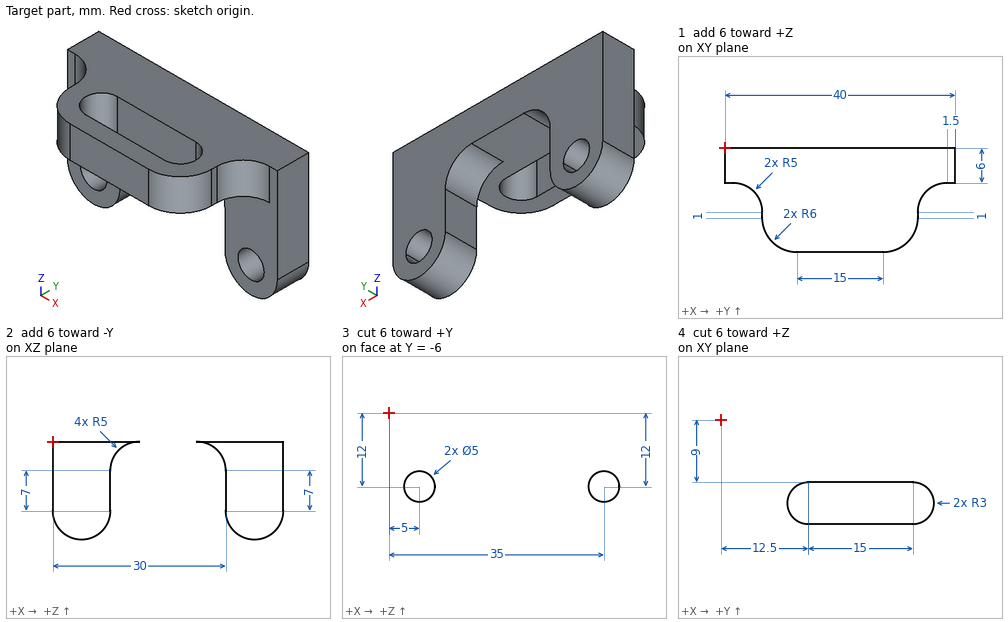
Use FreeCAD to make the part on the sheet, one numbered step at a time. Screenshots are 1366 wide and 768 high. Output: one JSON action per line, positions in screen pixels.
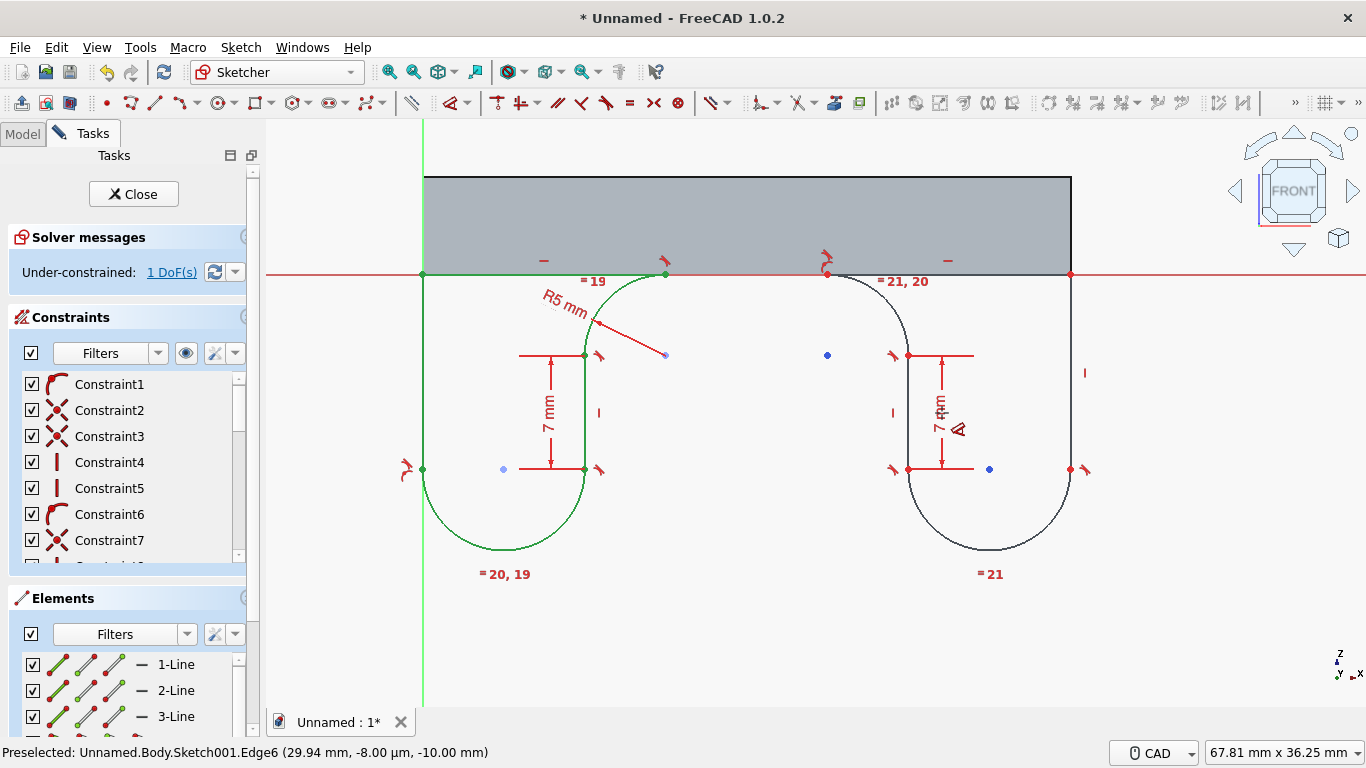
{"action": "left_click", "coordinate": [908, 469]}
{"action": "left_click", "coordinate": [665, 241]}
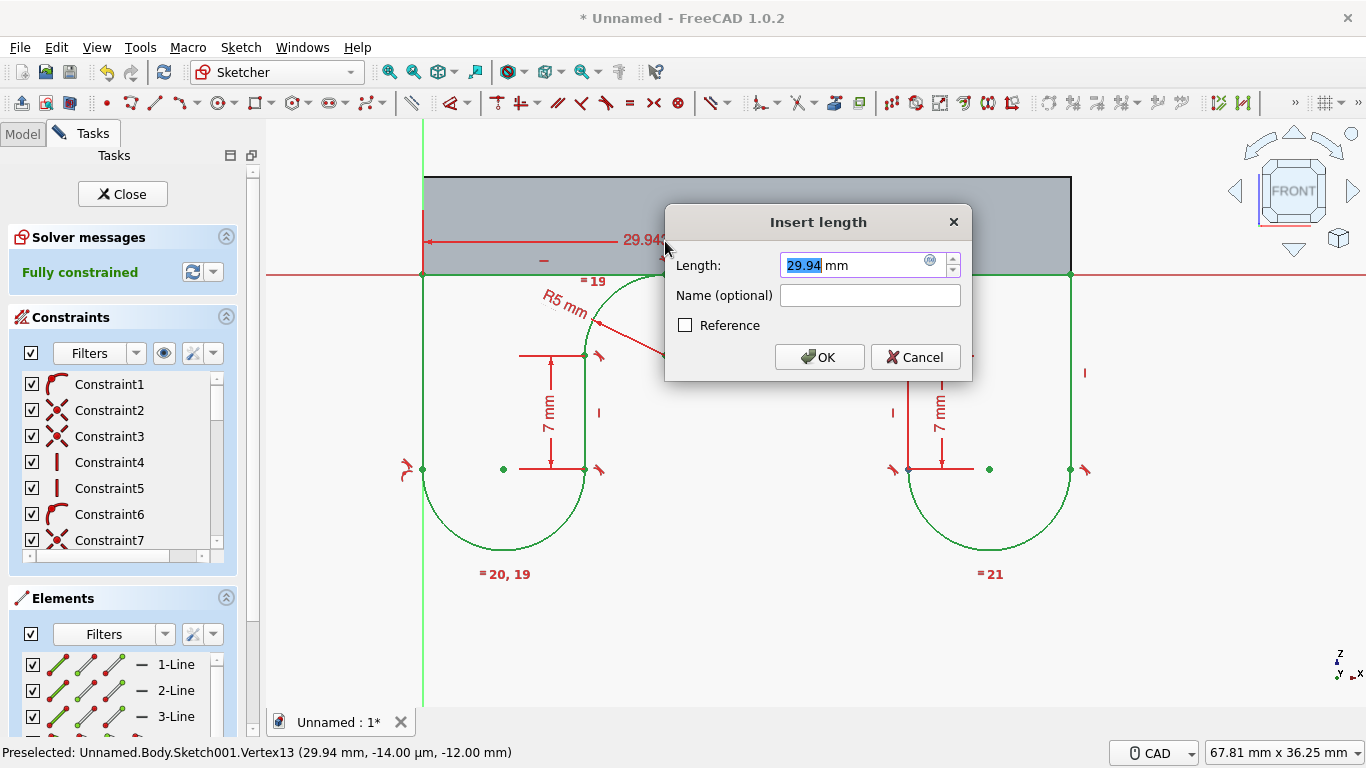
{"action": "type", "text": "30"}
{"action": "key", "text": "Return"}
{"action": "key", "text": "Escape"}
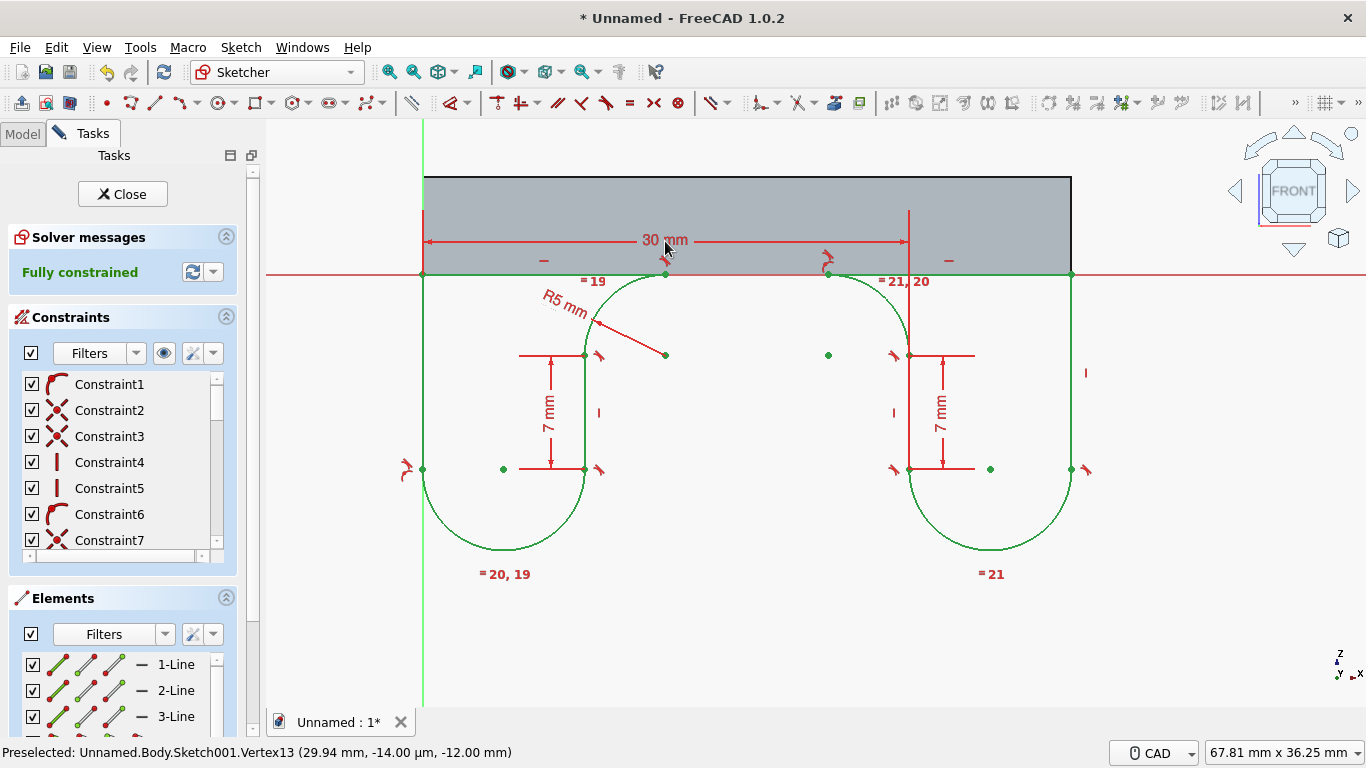
{"action": "left_click", "coordinate": [123, 194]}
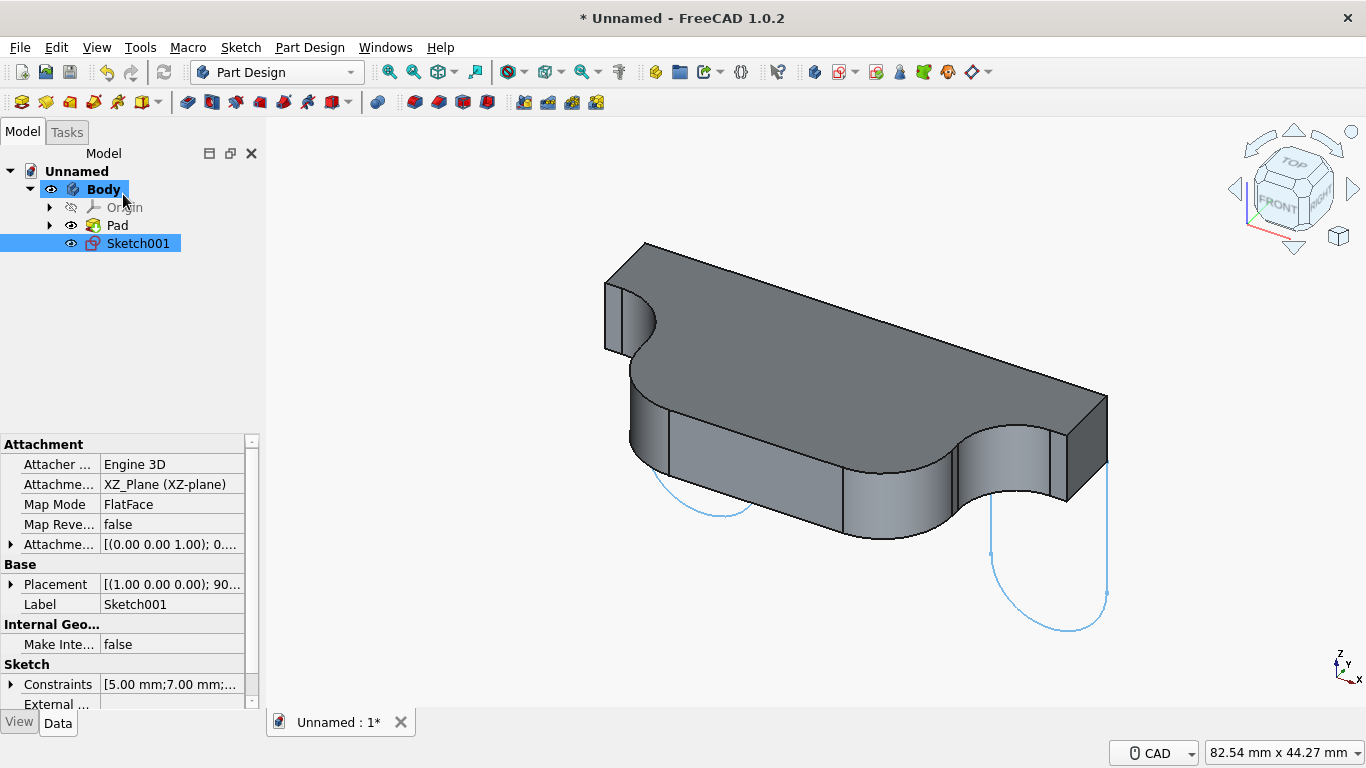
{"action": "left_click", "coordinate": [22, 102]}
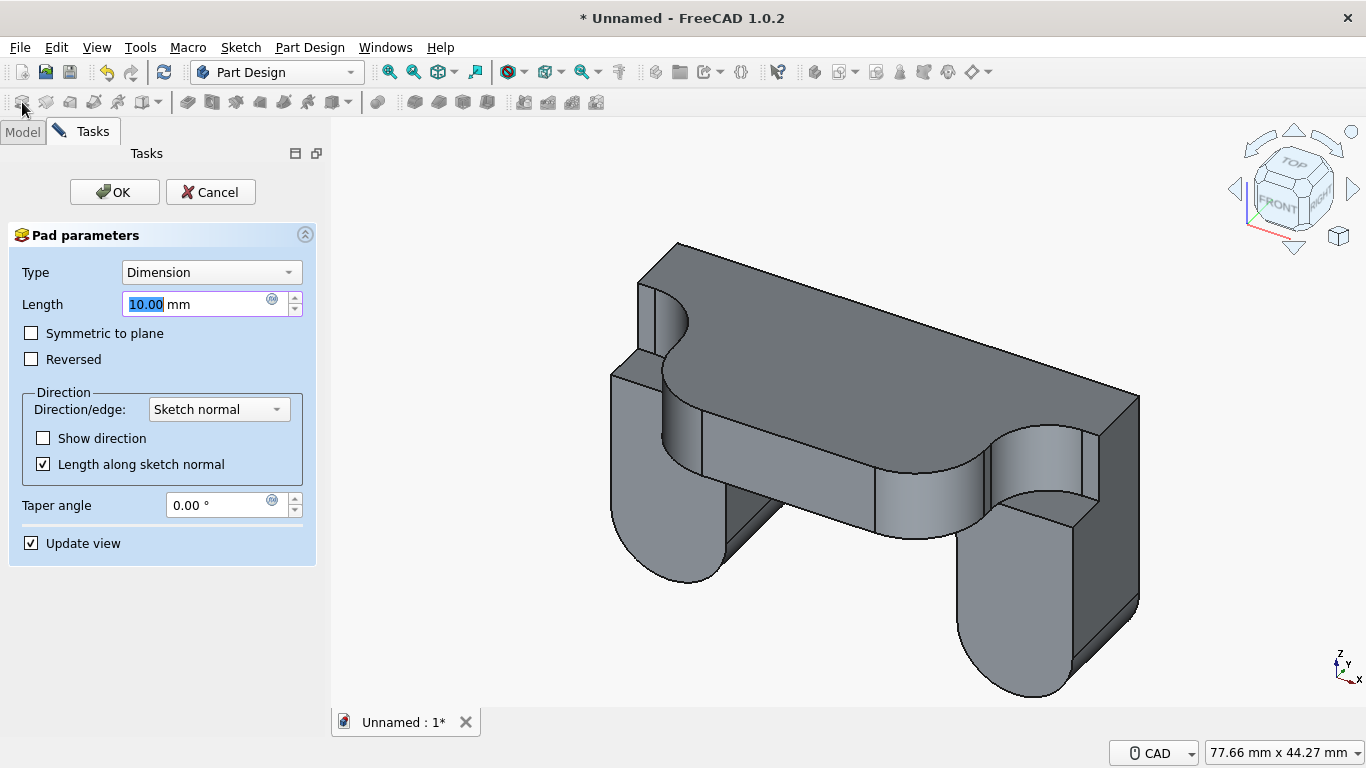
{"action": "type", "text": "6"}
{"action": "key", "text": "Tab"}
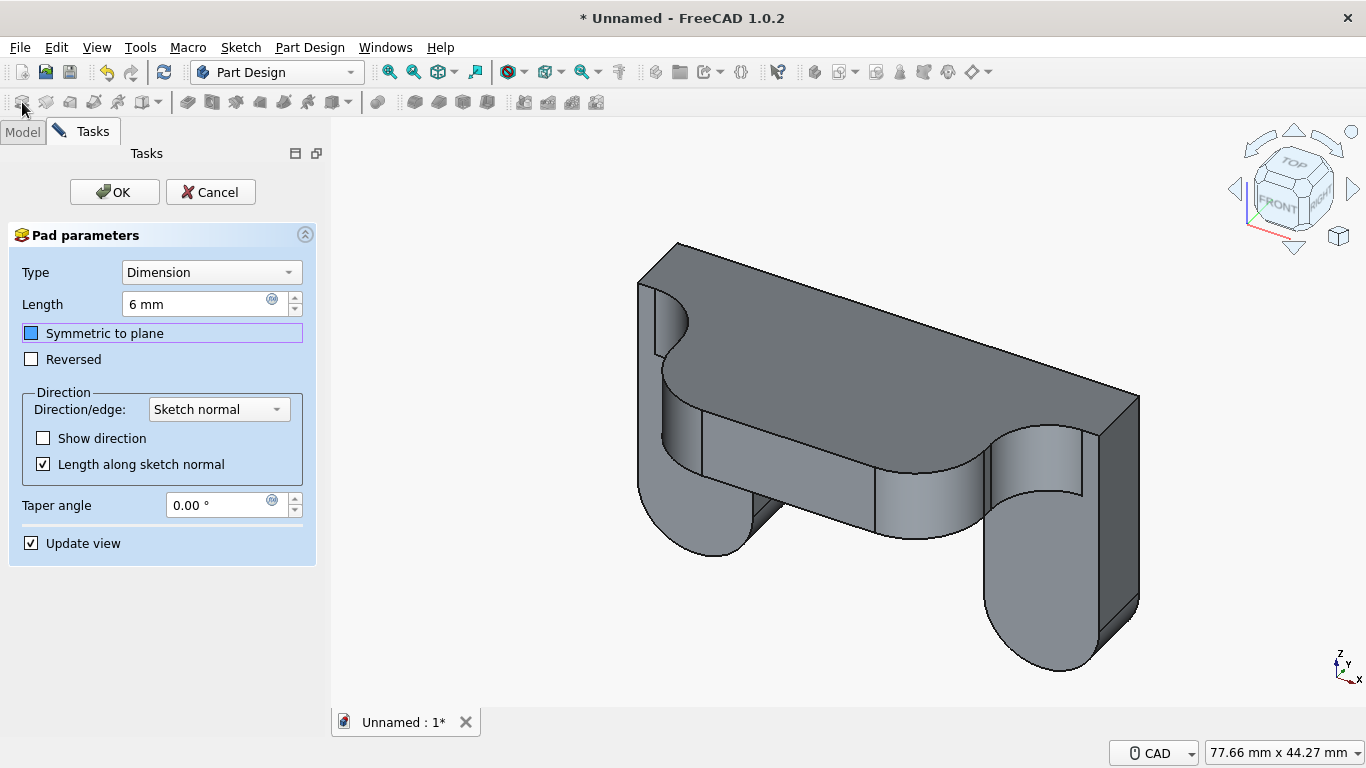
{"action": "left_click", "coordinate": [115, 192]}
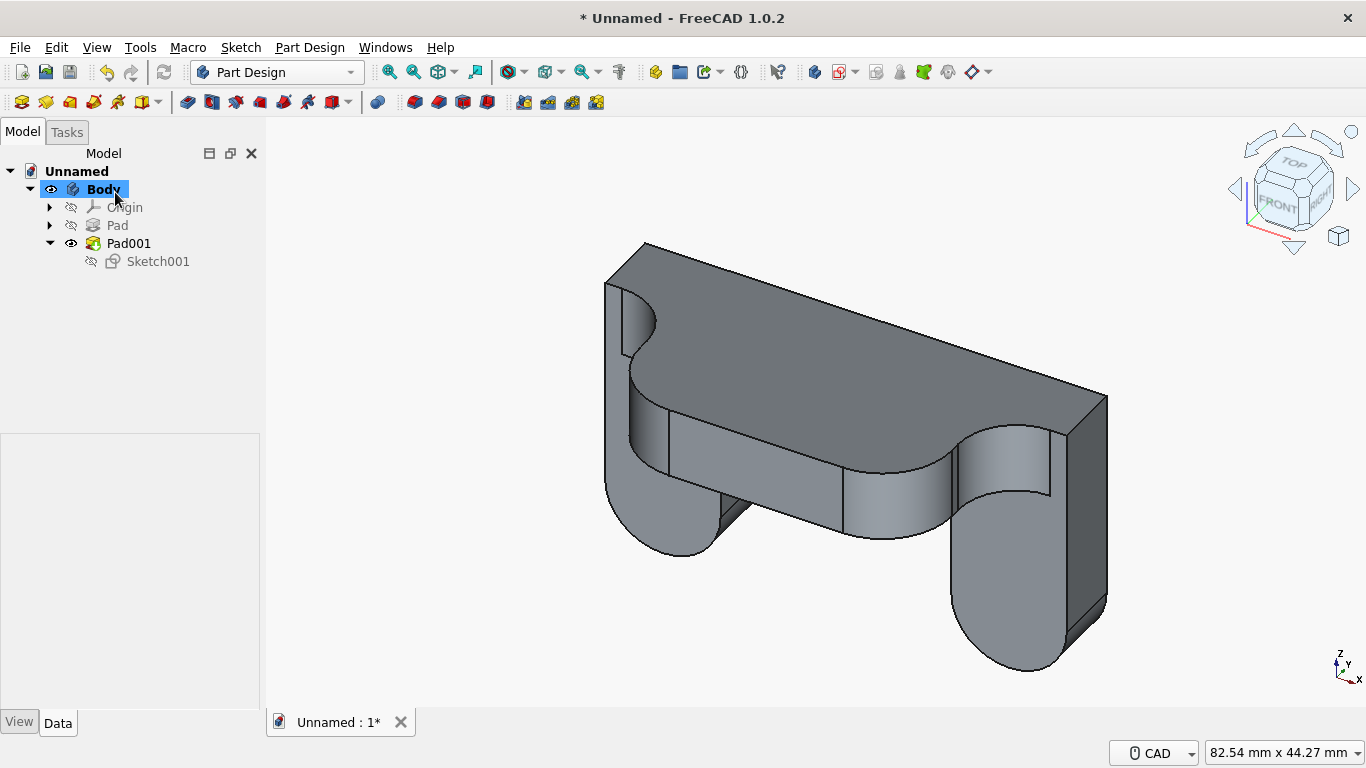
{"action": "left_click", "coordinate": [390, 72]}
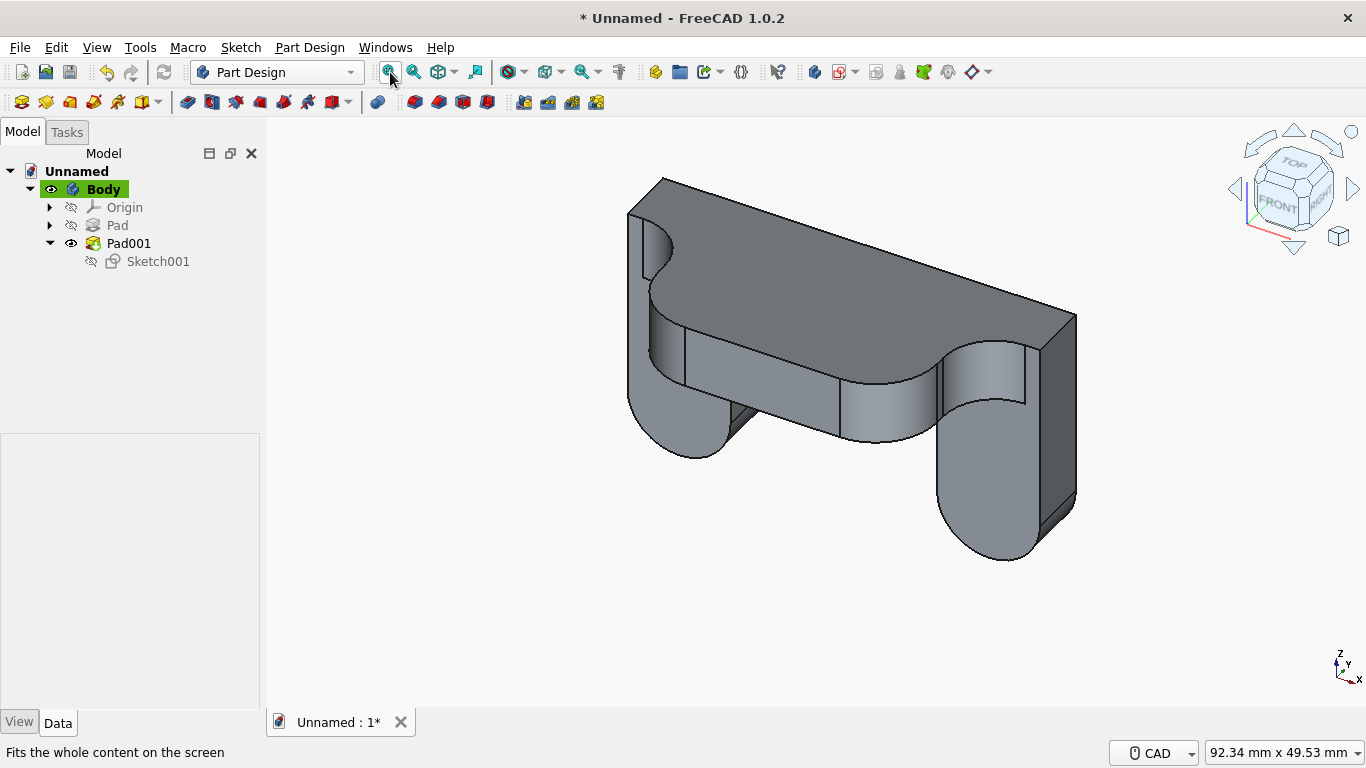
{"action": "left_click", "coordinate": [985, 443]}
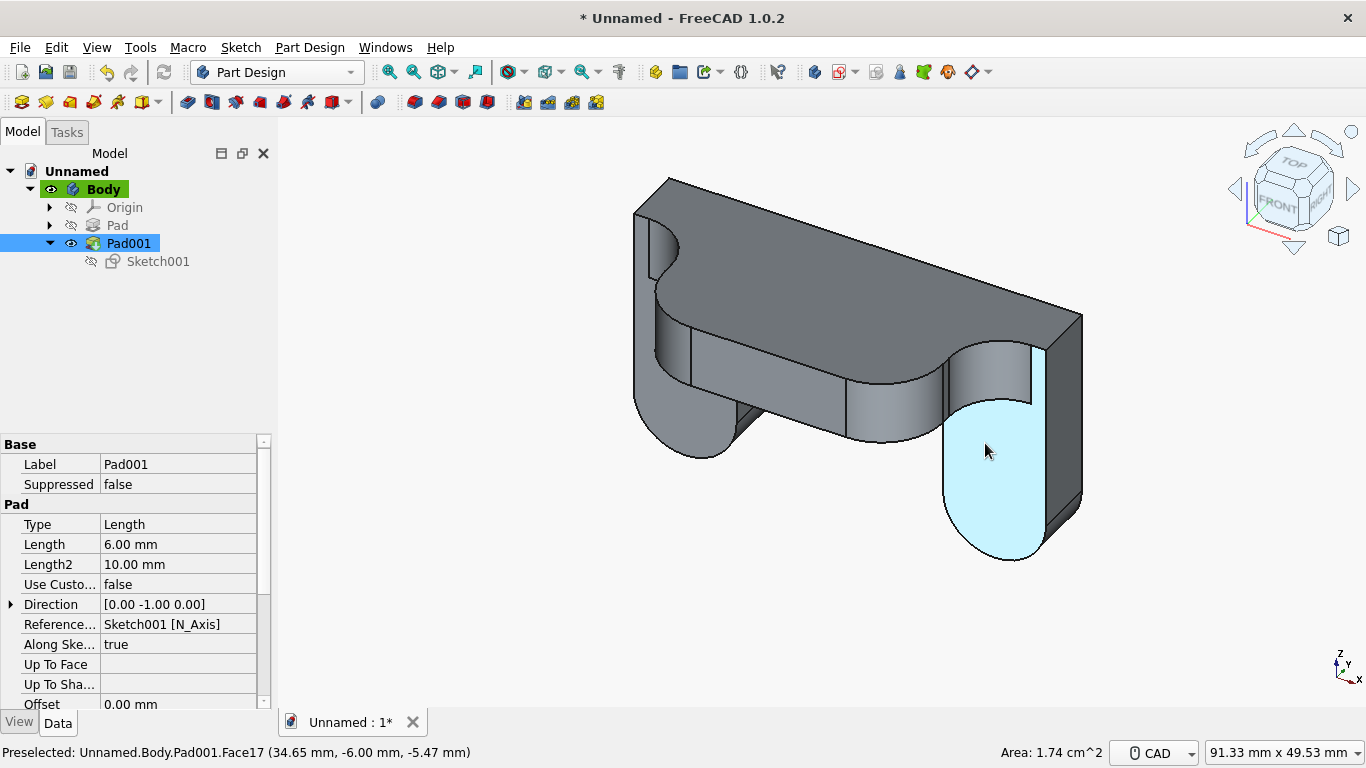
{"action": "left_click", "coordinate": [840, 72]}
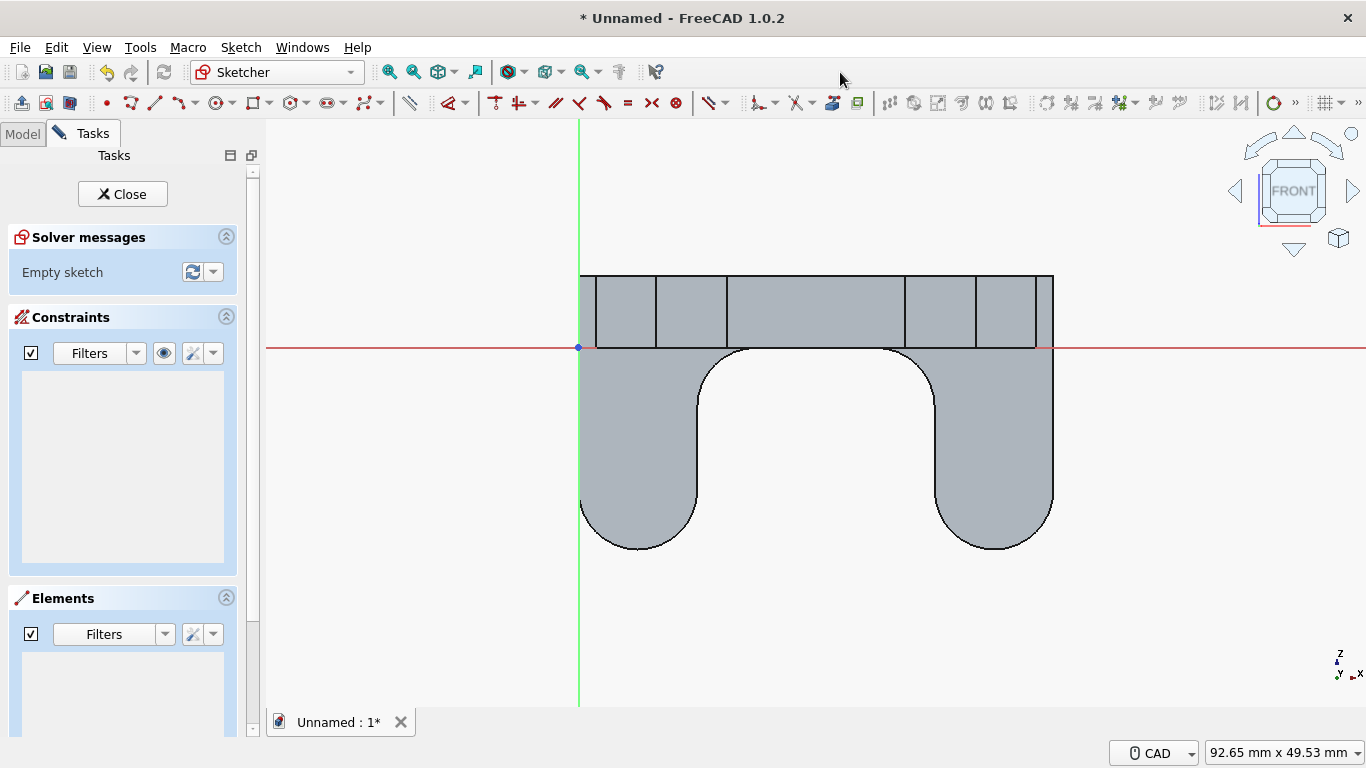
{"action": "scroll", "coordinate": [910, 476], "scroll_direction": "up", "scroll_amount": 2}